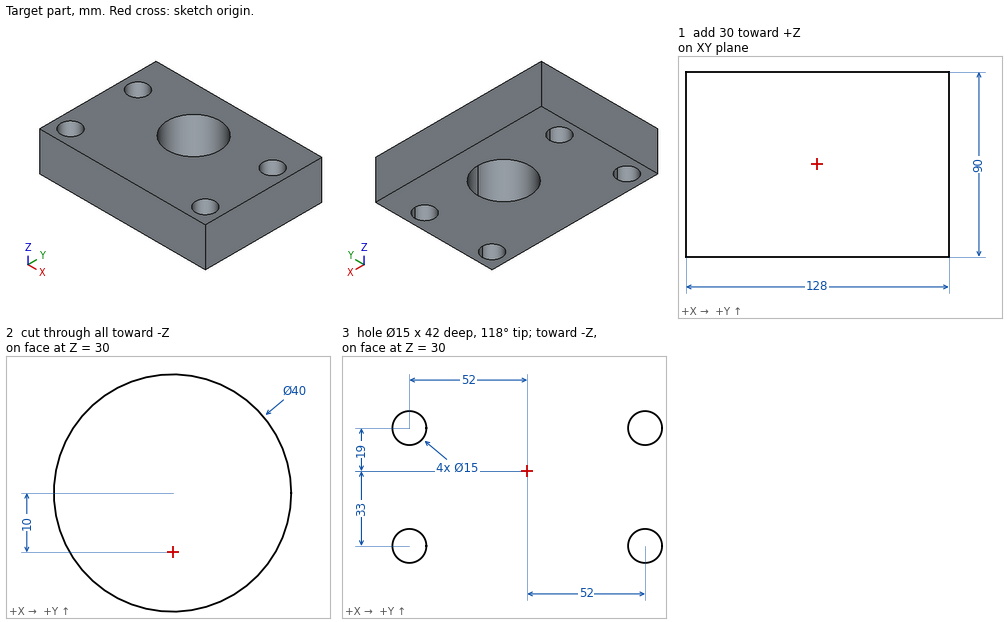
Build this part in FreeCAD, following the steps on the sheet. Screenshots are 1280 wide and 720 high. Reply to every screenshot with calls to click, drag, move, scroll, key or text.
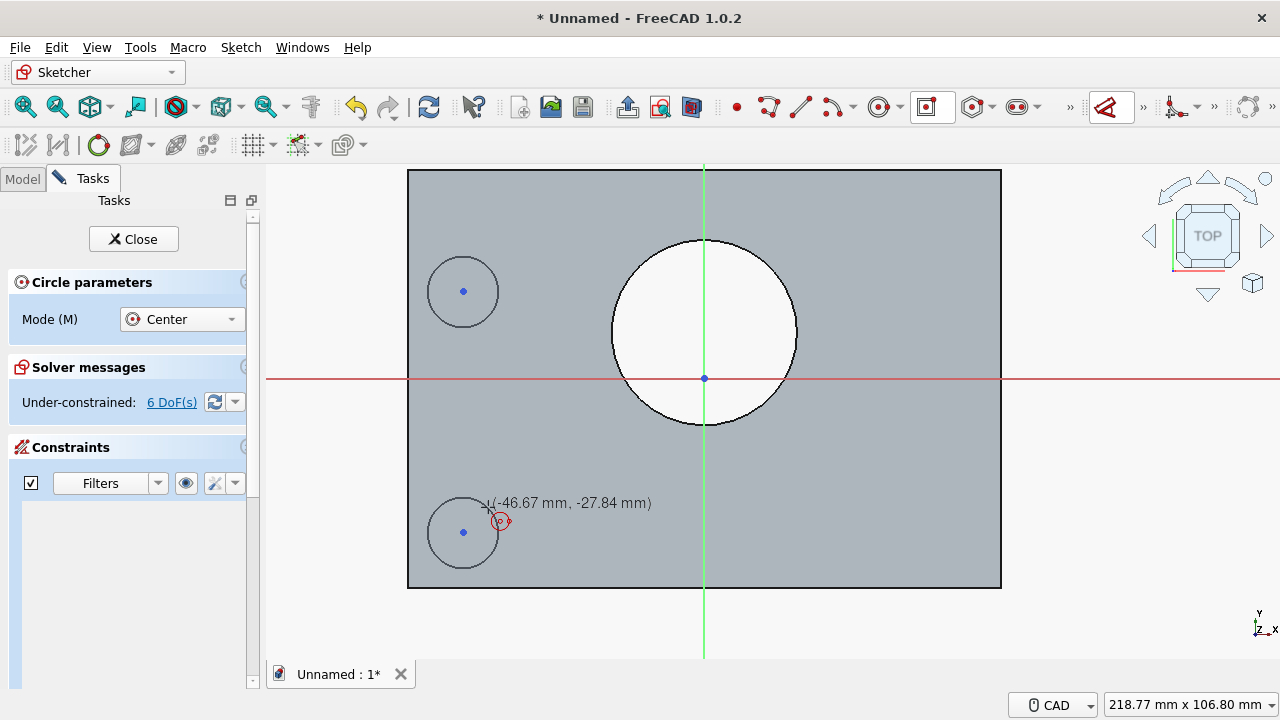
click(945, 532)
click(970, 507)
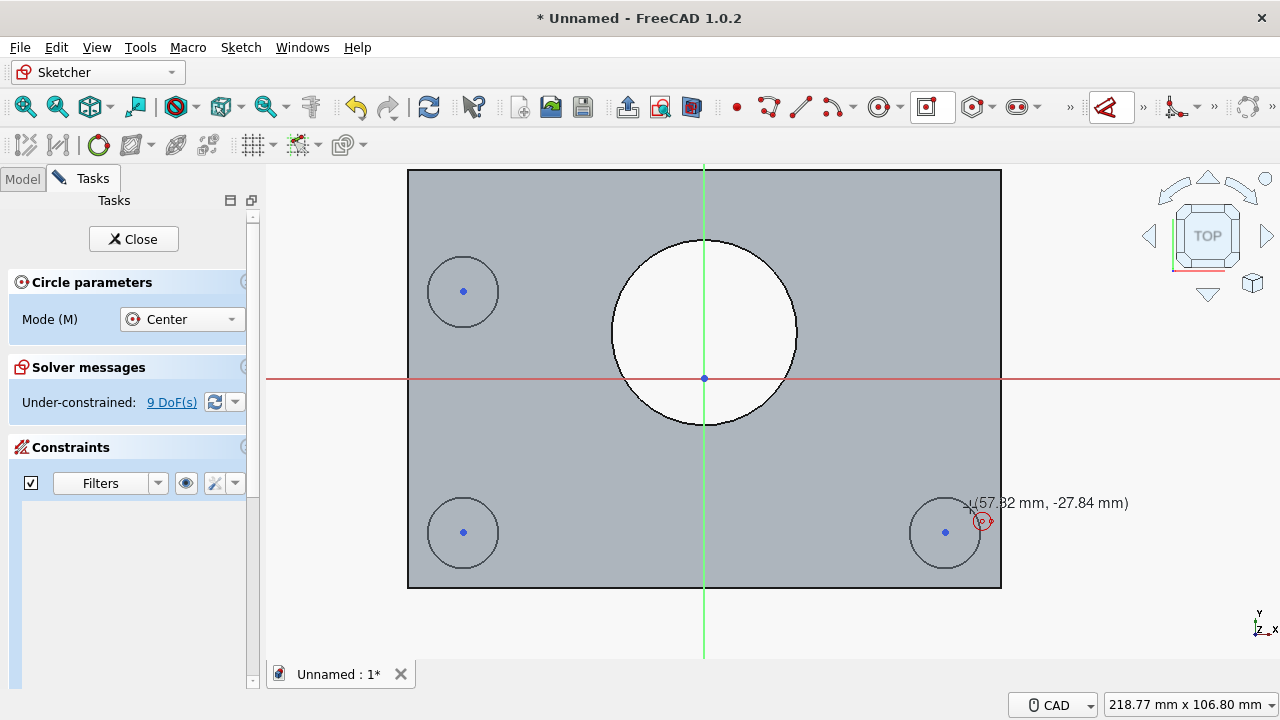
click(945, 291)
click(970, 266)
key(Escape)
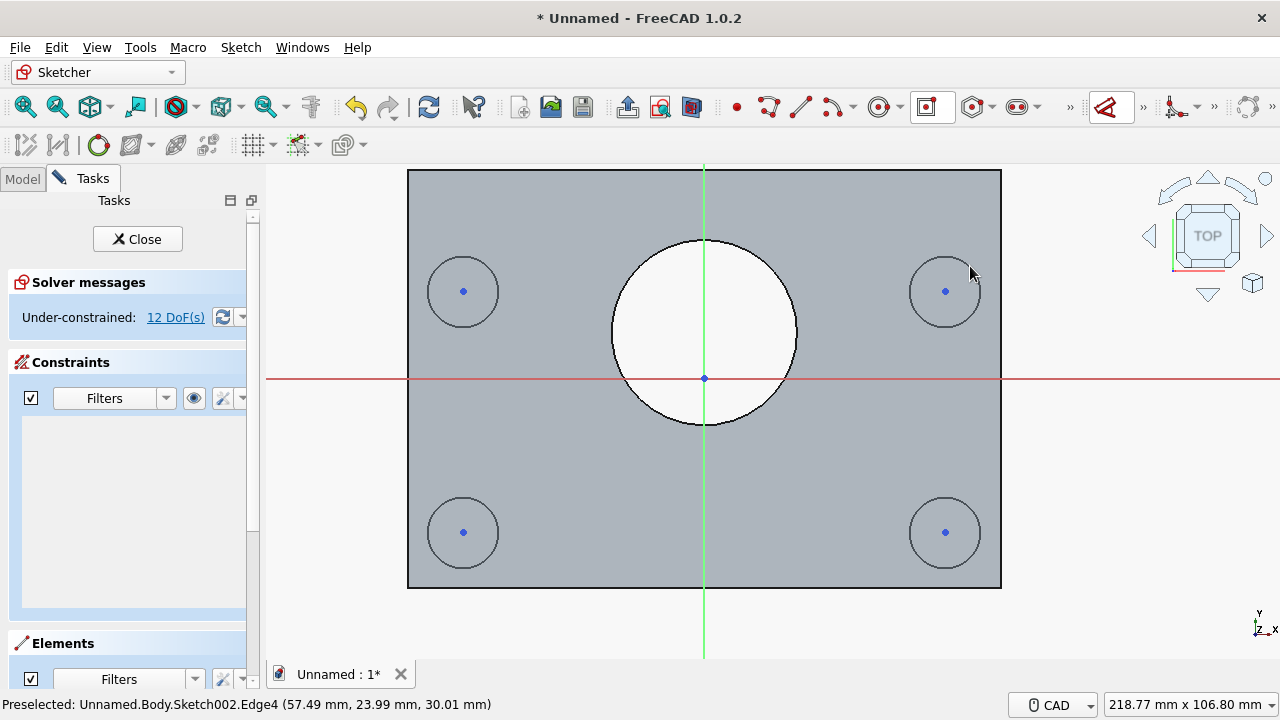
click(488, 267)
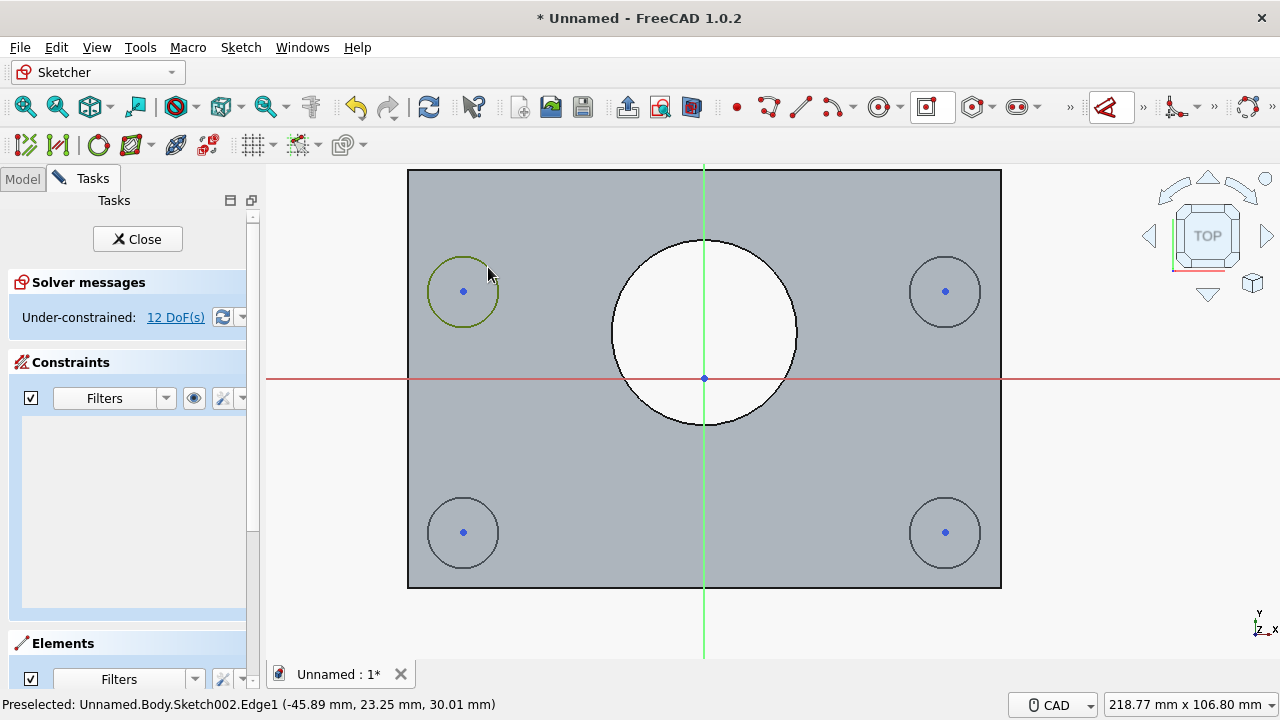
click(488, 508)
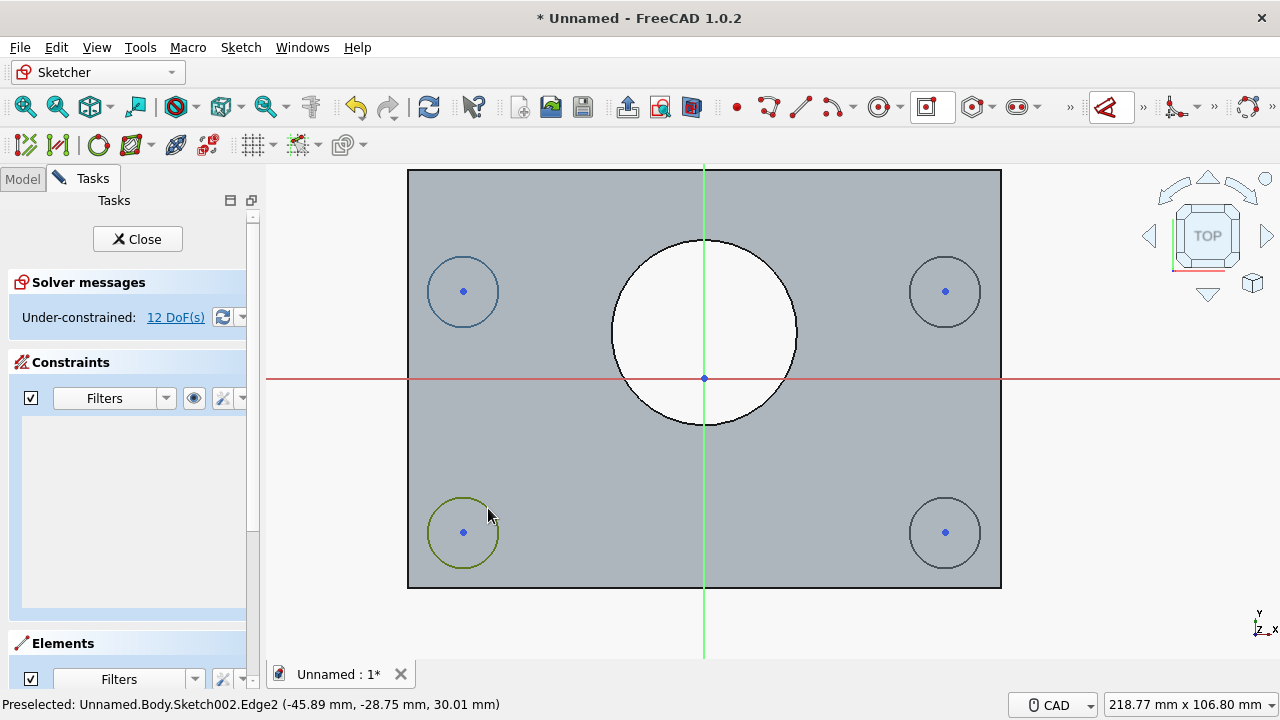
click(970, 508)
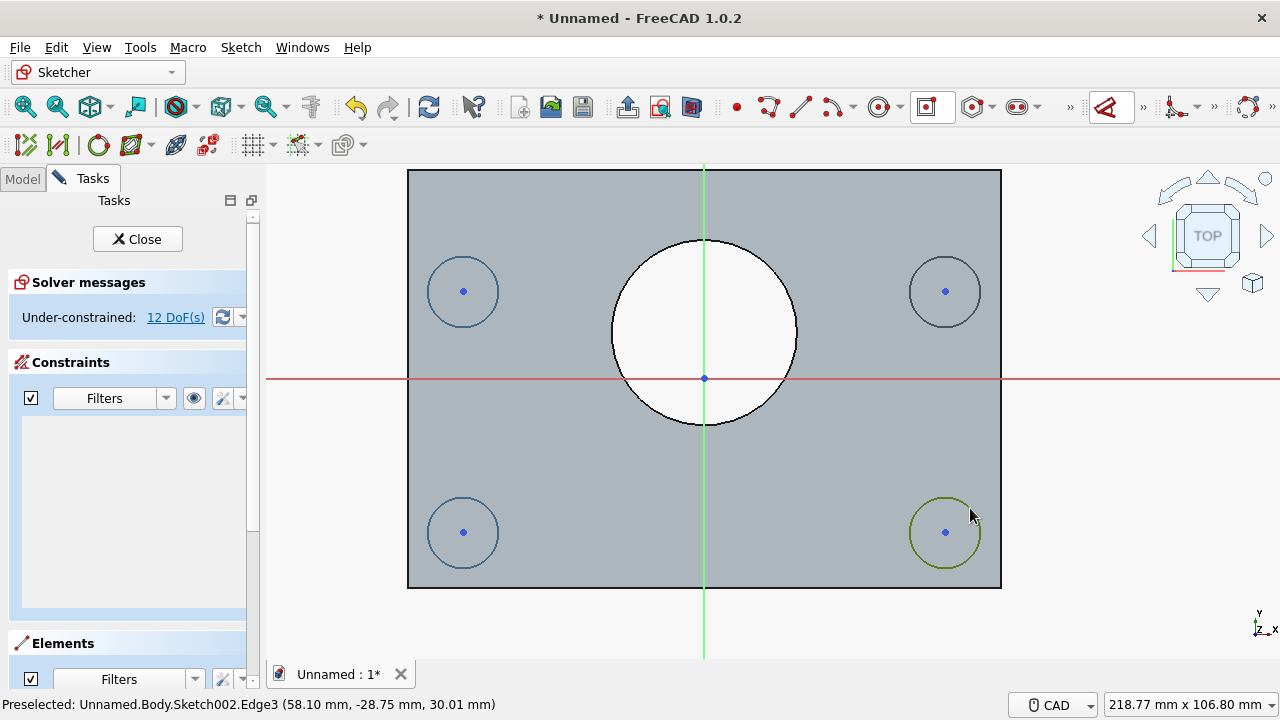
click(970, 267)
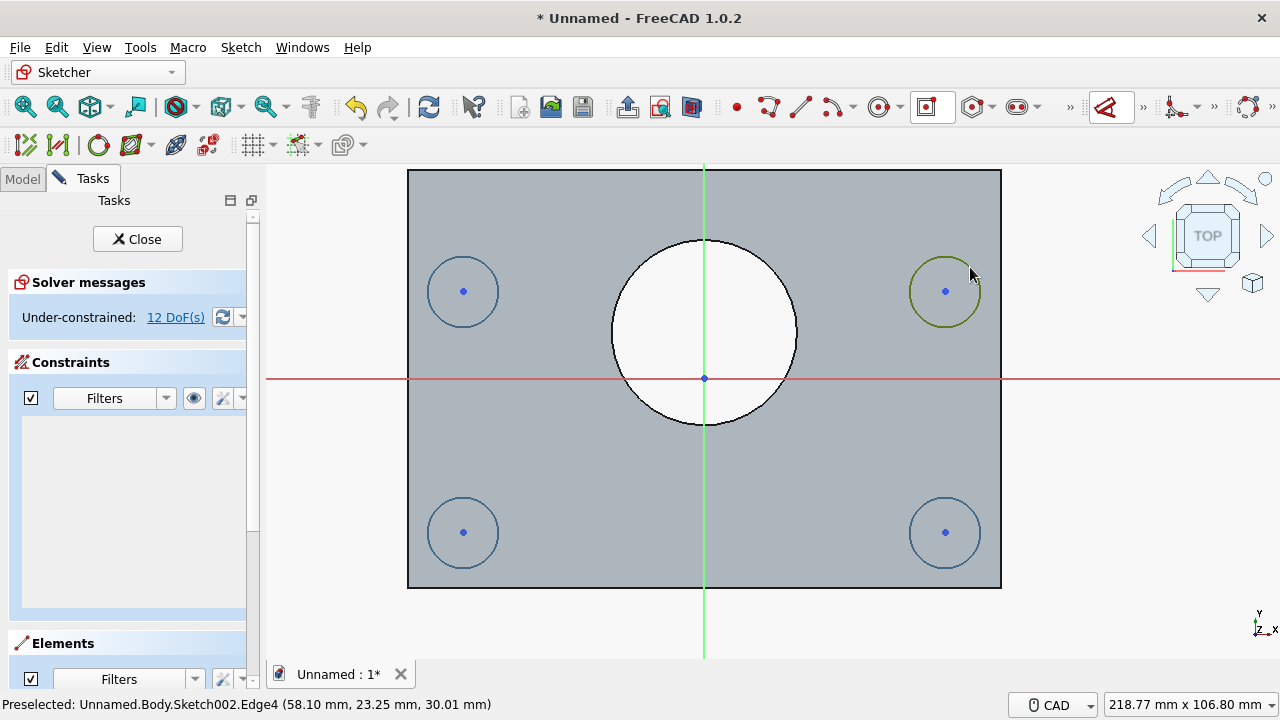
key(e)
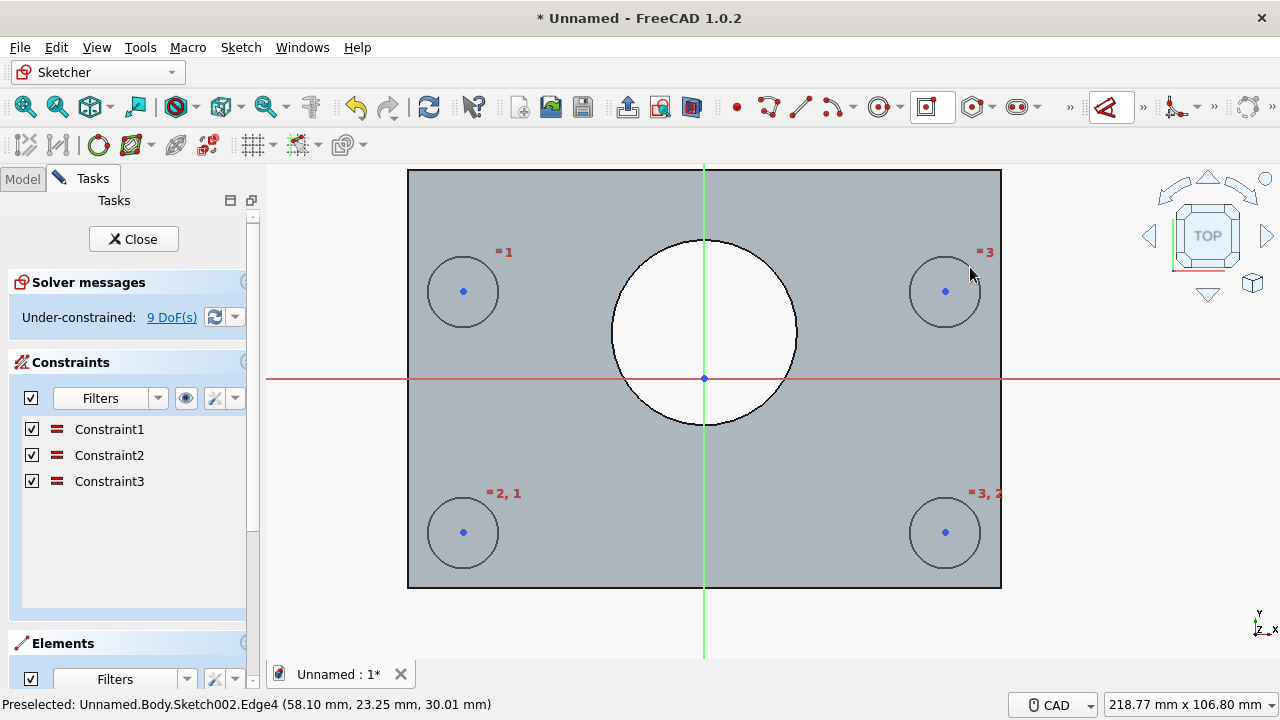
click(463, 292)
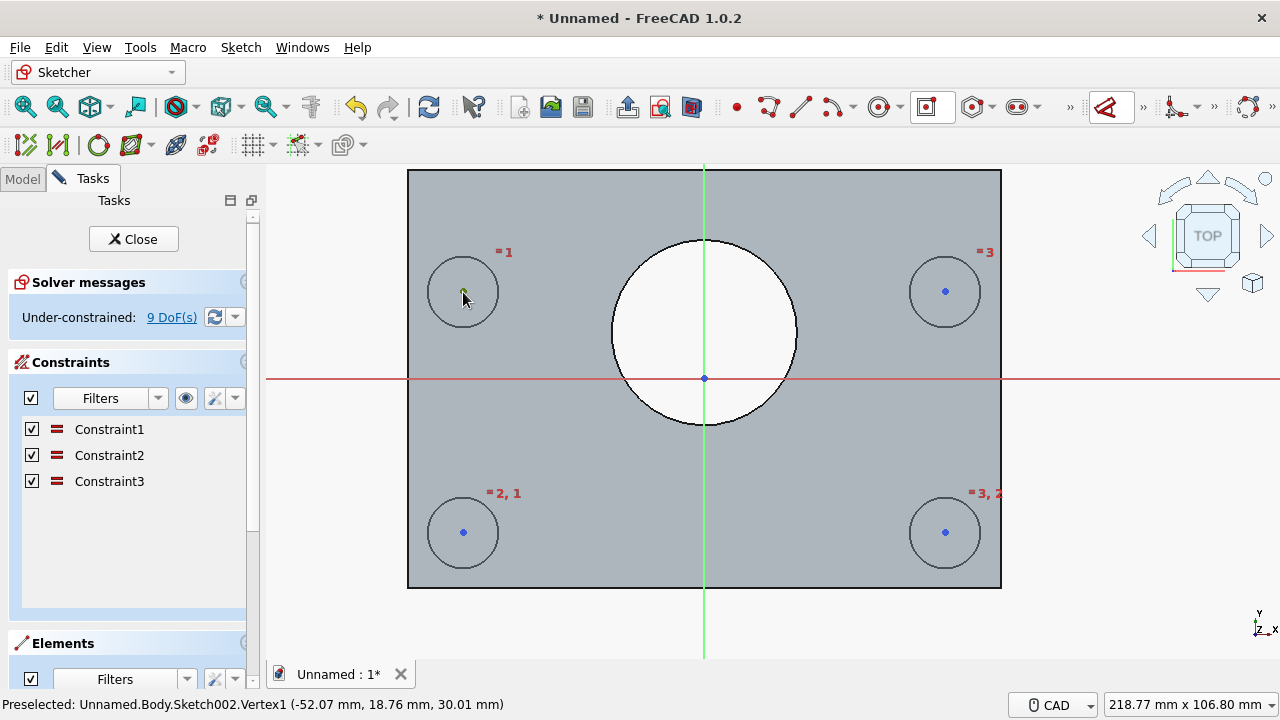
click(463, 533)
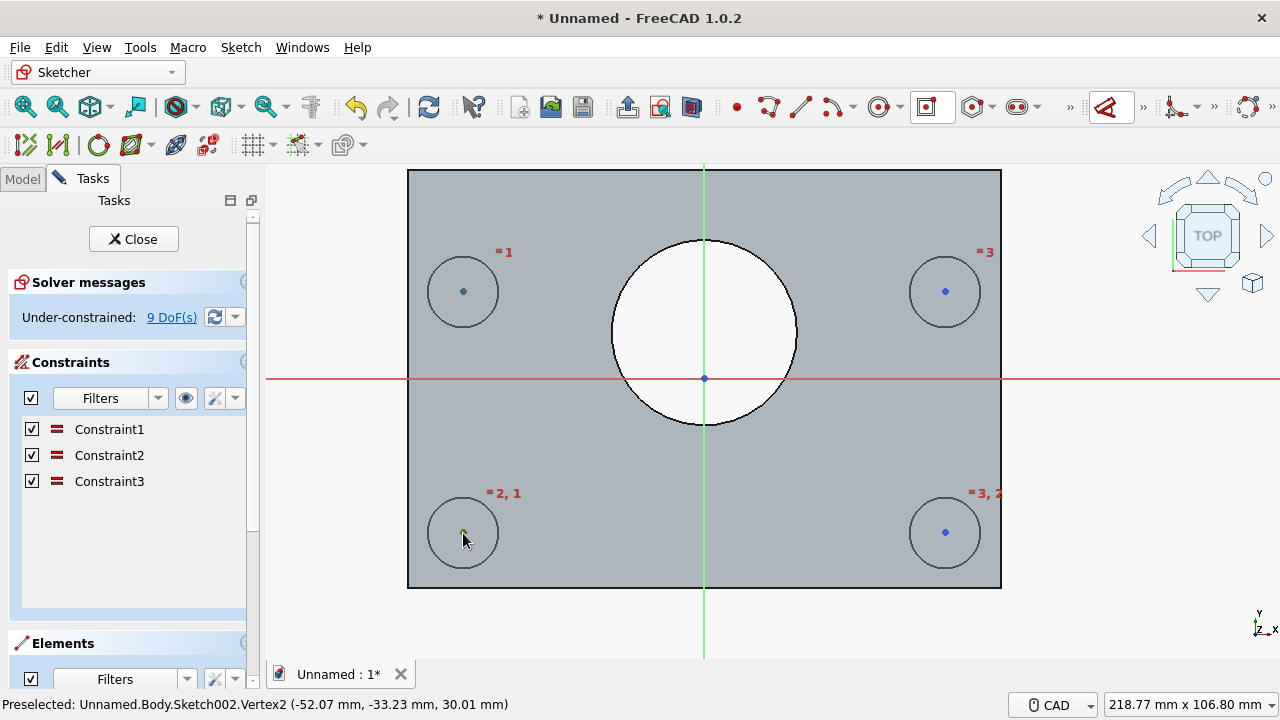
key(v)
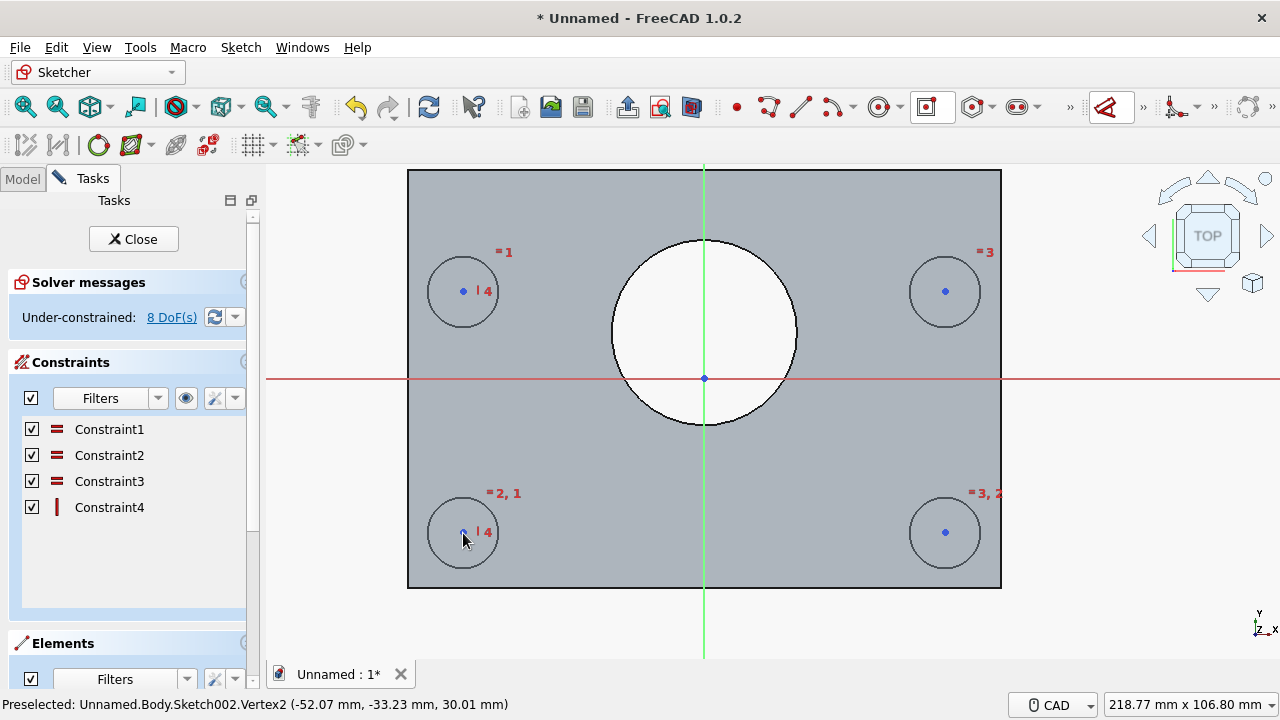
click(463, 533)